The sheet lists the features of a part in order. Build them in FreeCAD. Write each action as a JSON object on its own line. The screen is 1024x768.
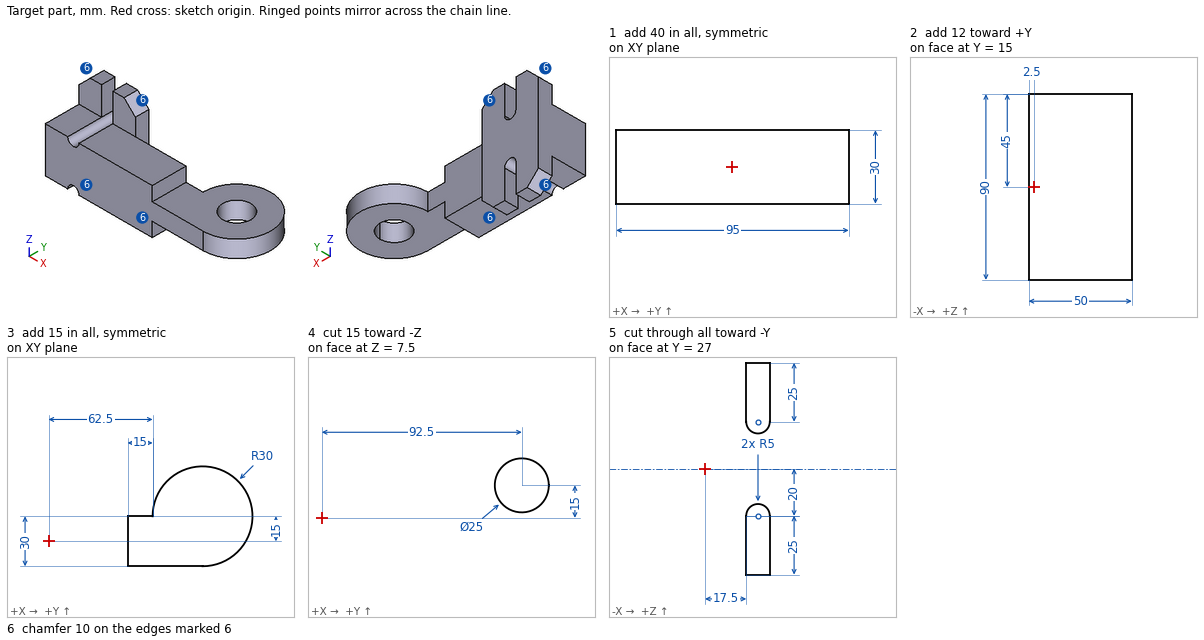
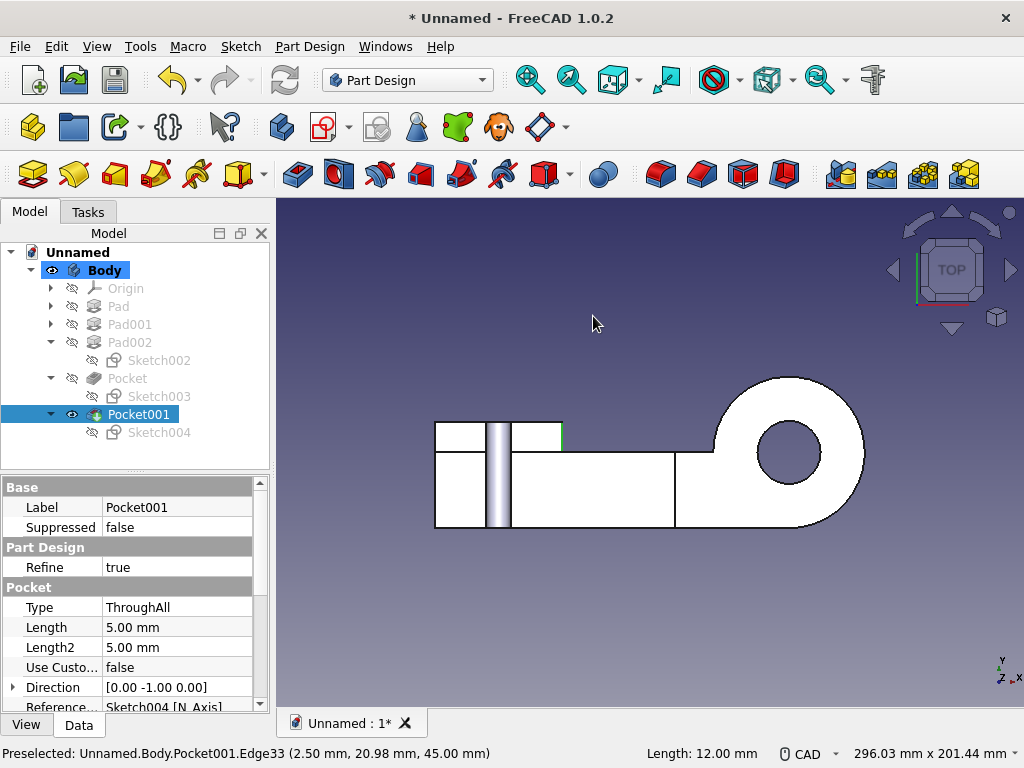
{"action": "left_click", "coordinate": [435, 436], "text": "ctrl"}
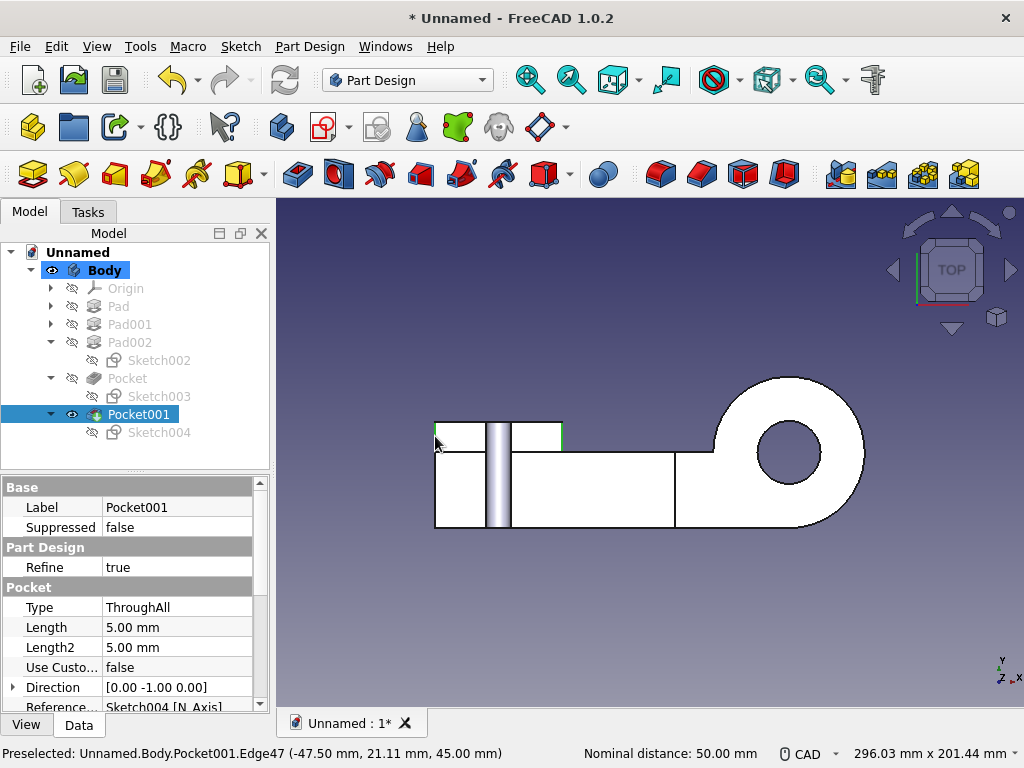
{"action": "key", "text": "1"}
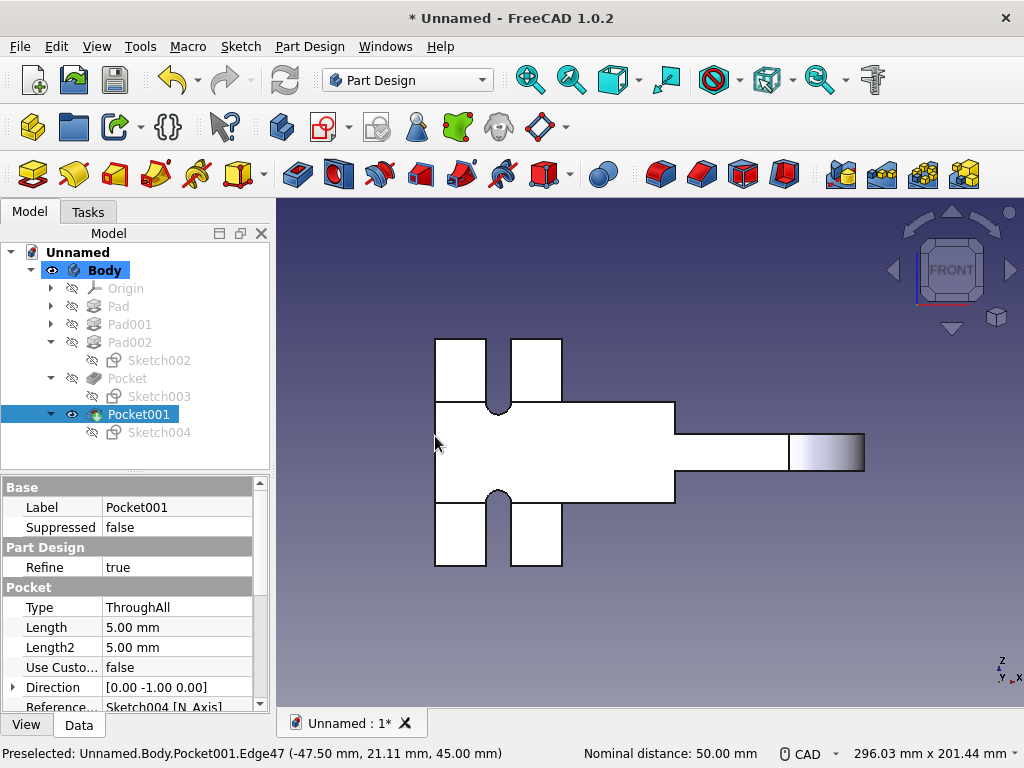
{"action": "key", "text": "3"}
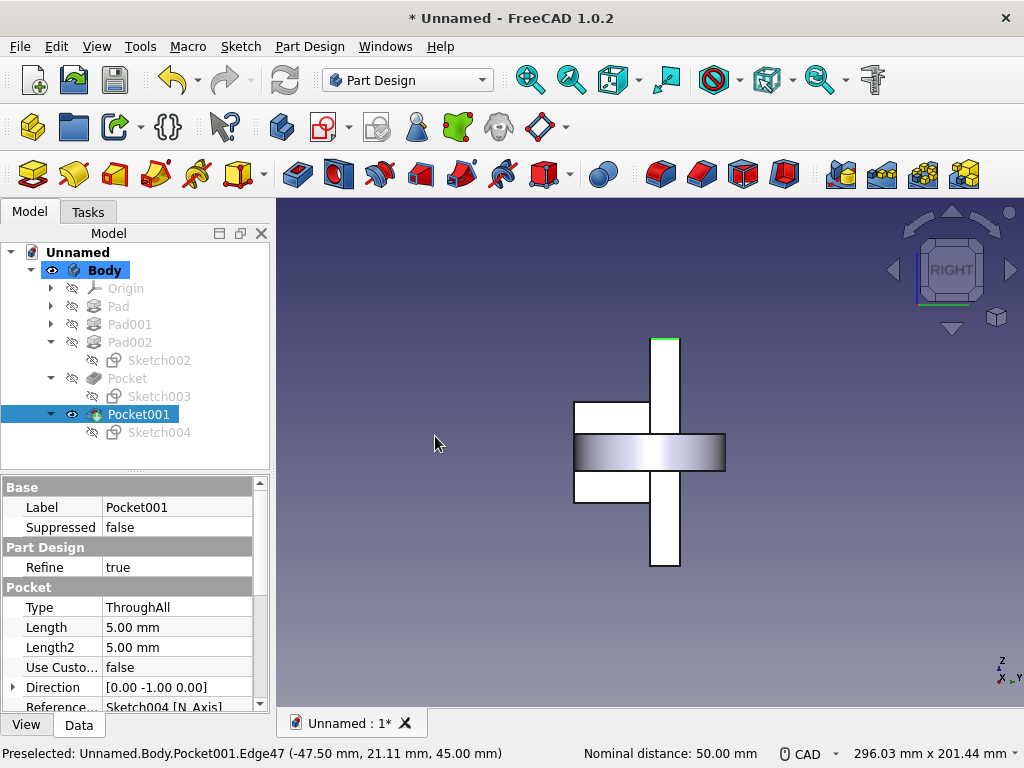
{"action": "left_click", "coordinate": [531, 80]}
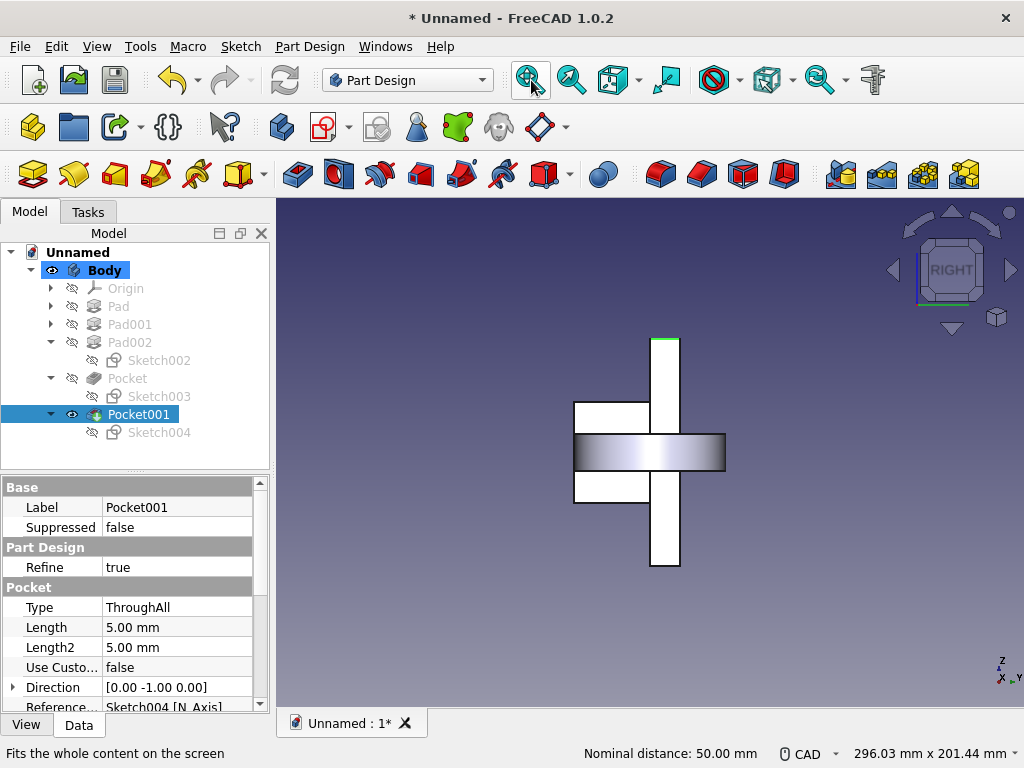
{"action": "left_click", "coordinate": [665, 565], "text": "ctrl"}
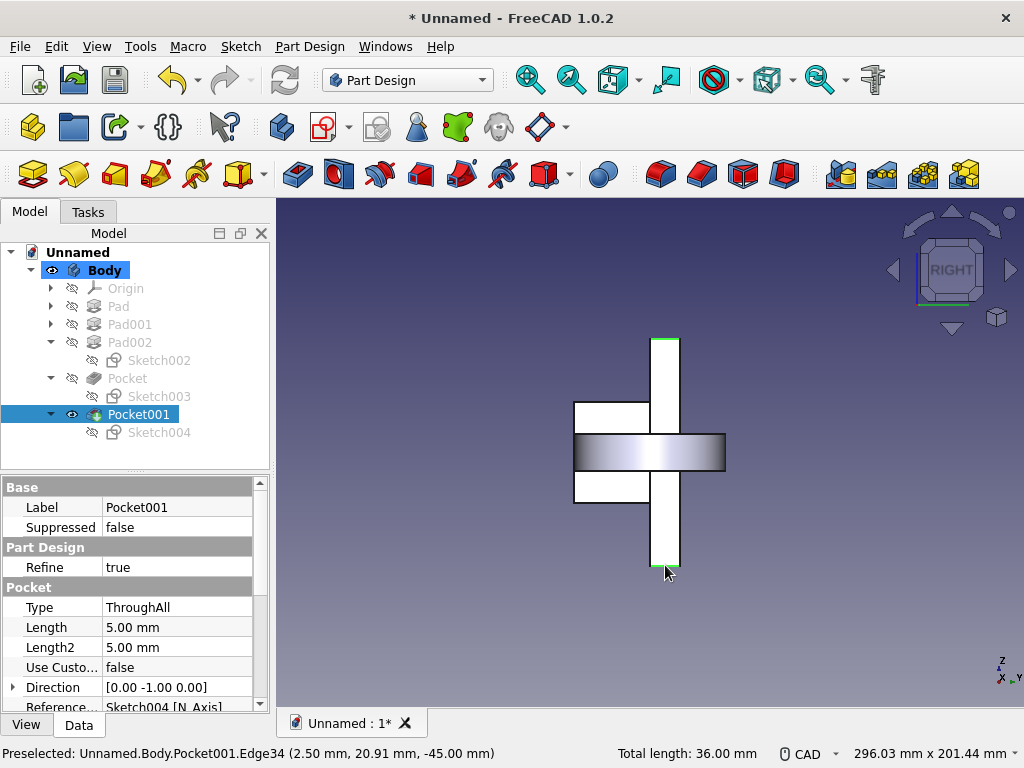
{"action": "key", "text": "5"}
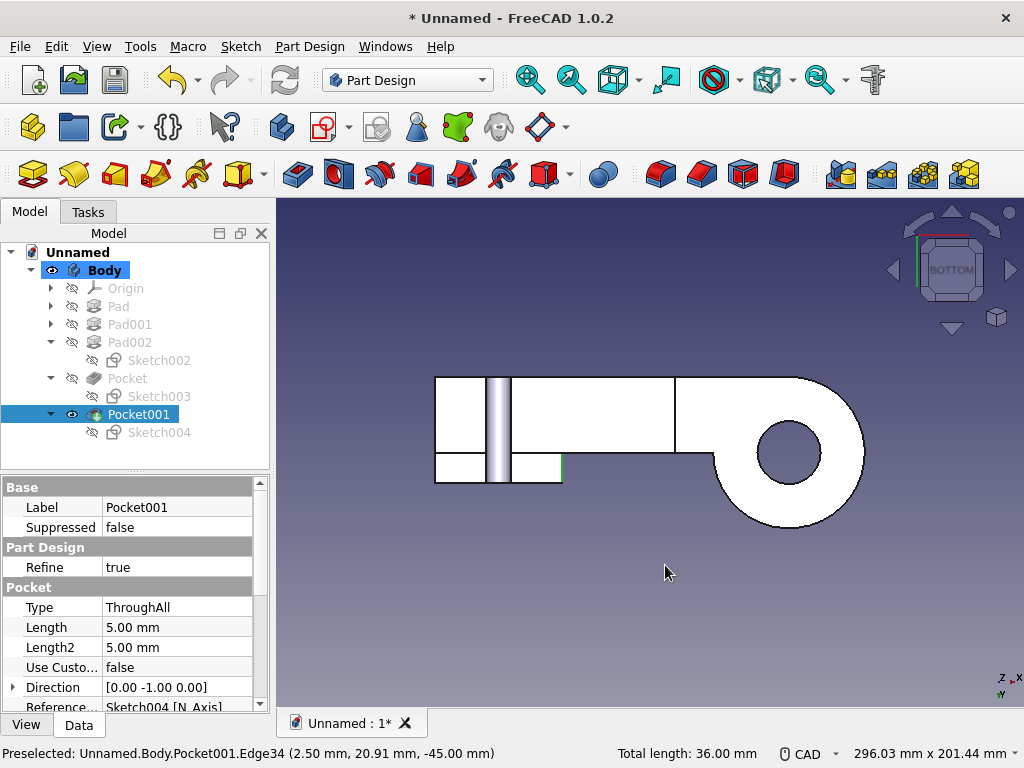
{"action": "left_click", "coordinate": [435, 467], "text": "ctrl"}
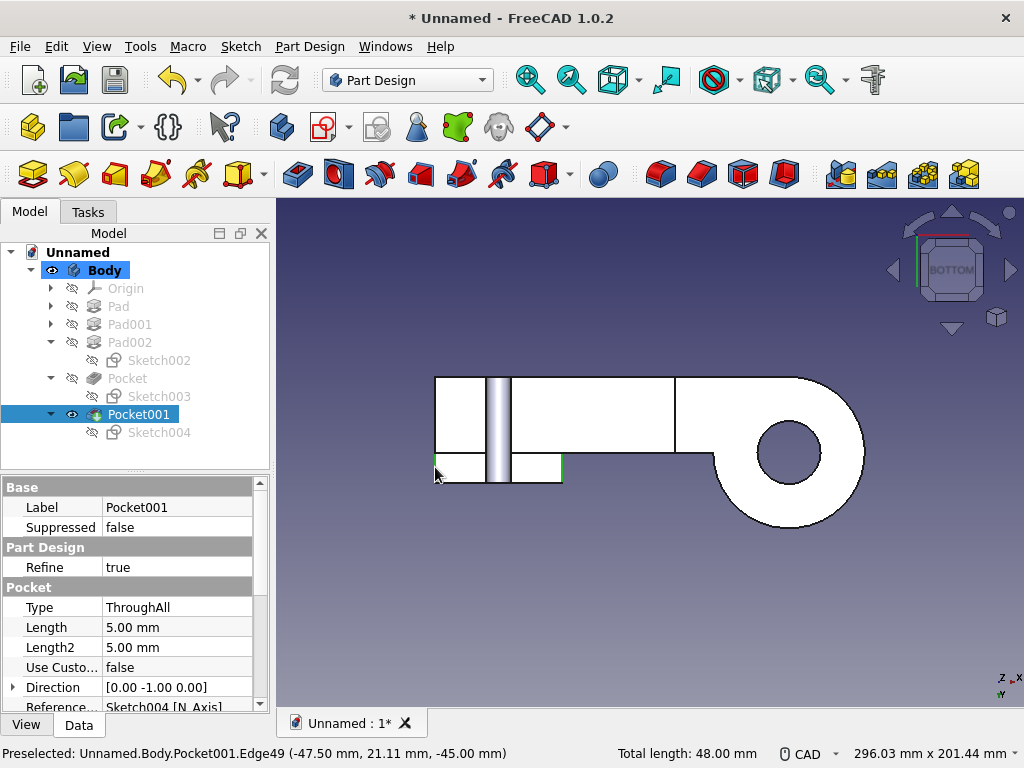
{"action": "left_click", "coordinate": [702, 174]}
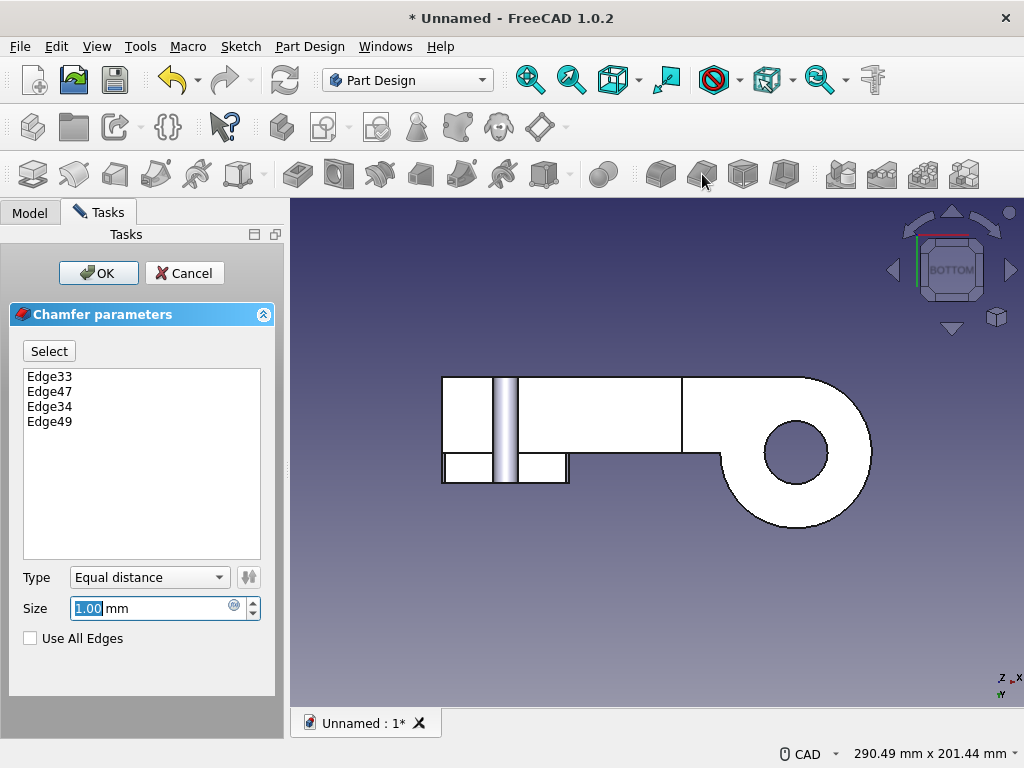
{"action": "type", "text": "10"}
{"action": "key", "text": "Tab"}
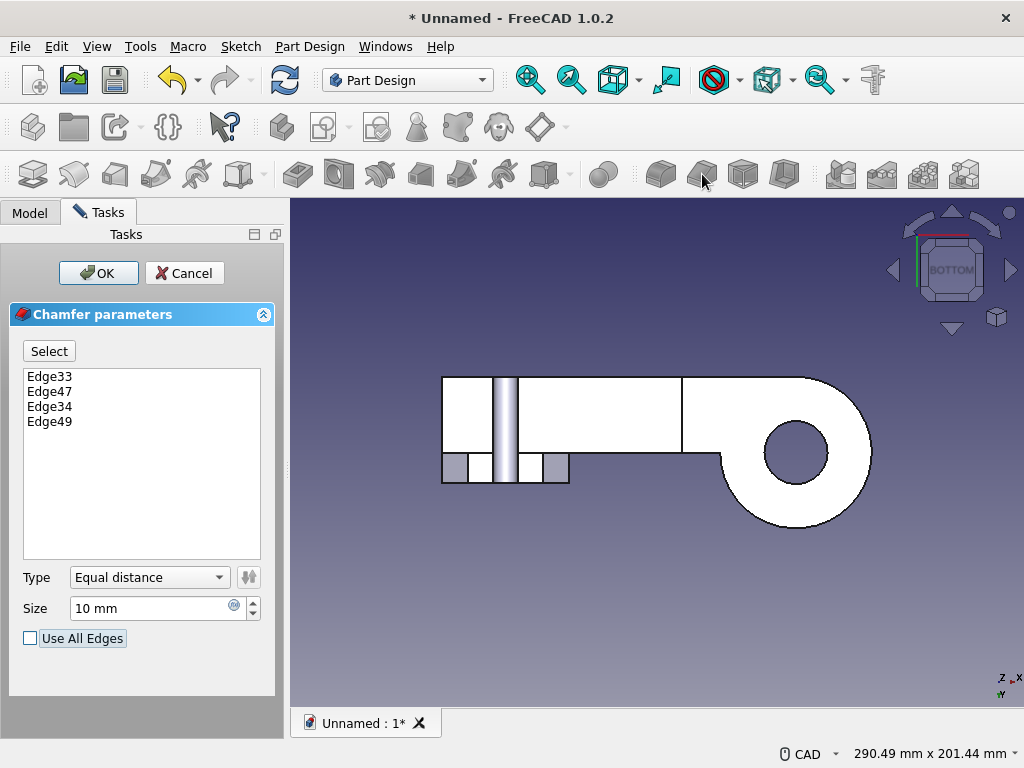
{"action": "left_click", "coordinate": [99, 273]}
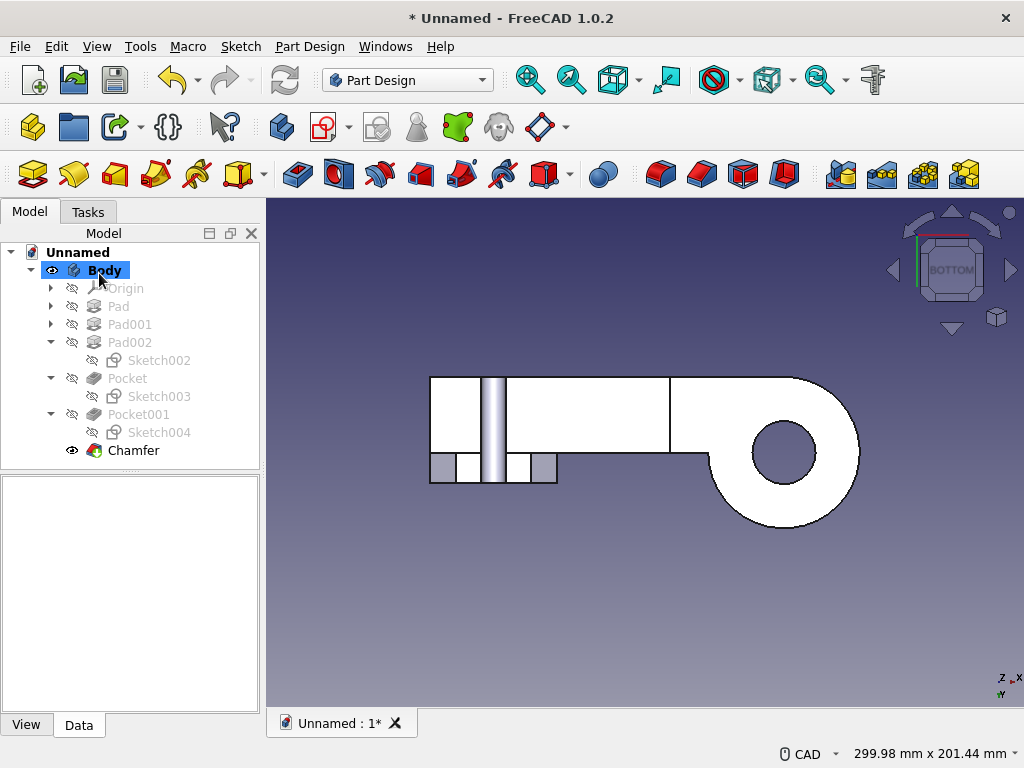
{"action": "key", "text": "0"}